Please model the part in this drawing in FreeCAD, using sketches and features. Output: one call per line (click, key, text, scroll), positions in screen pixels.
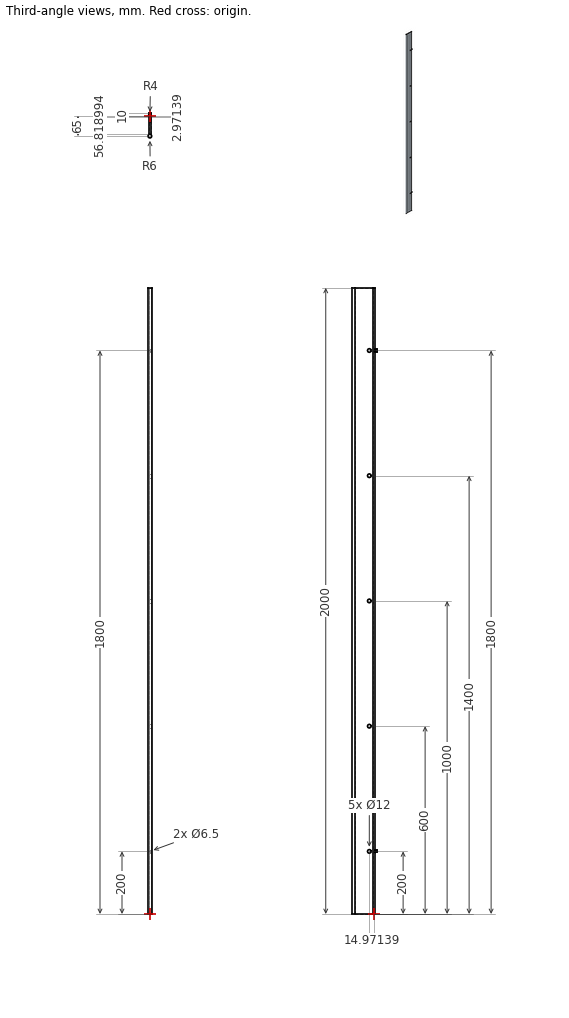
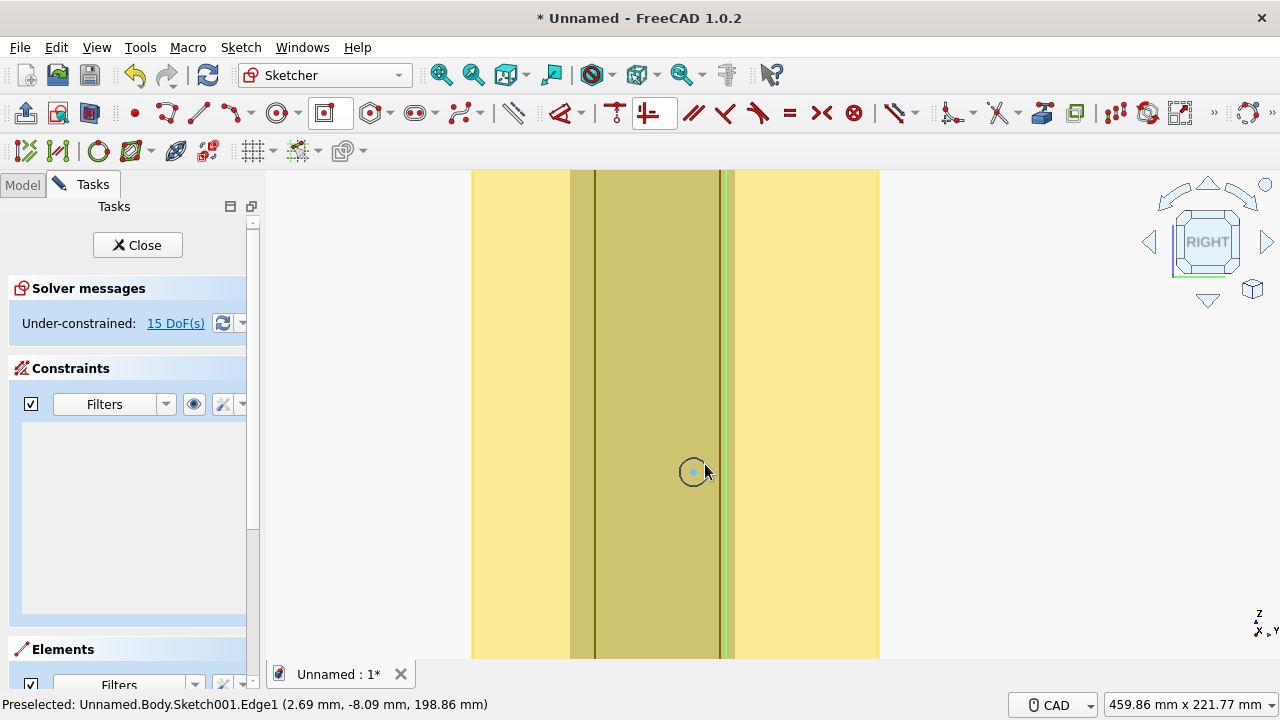
click(703, 462)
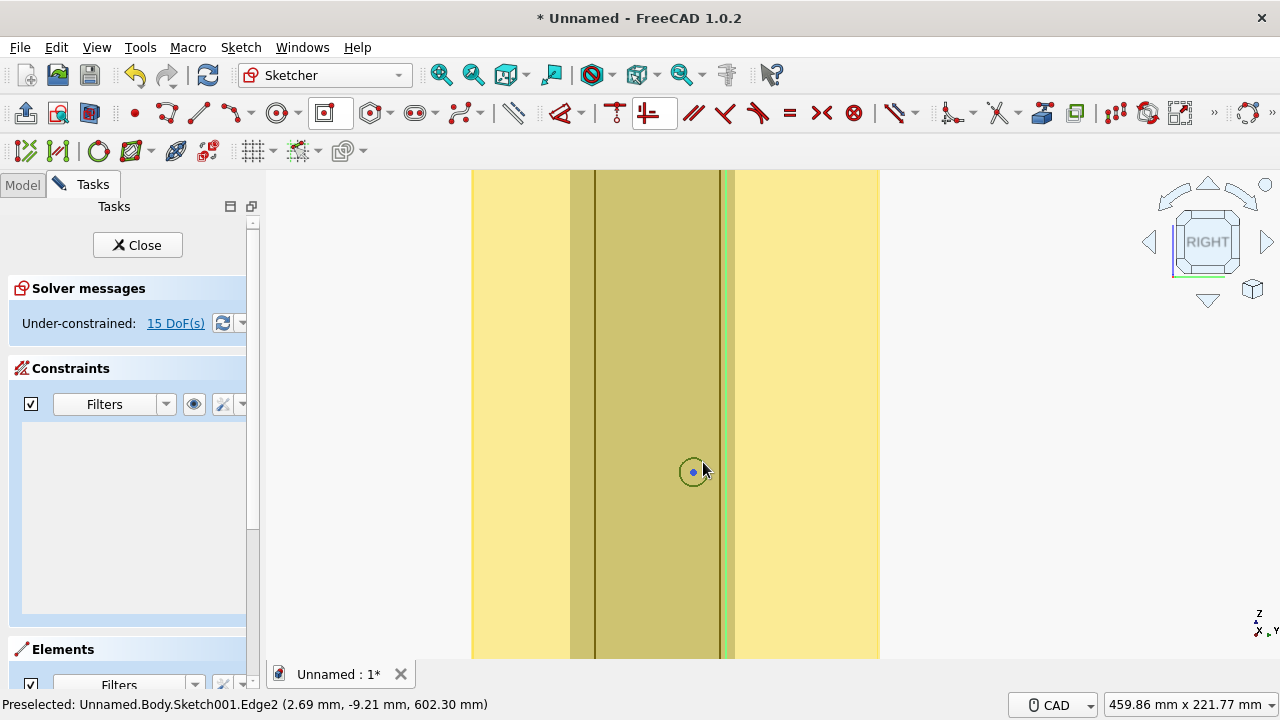
scroll(705, 464, down, 13)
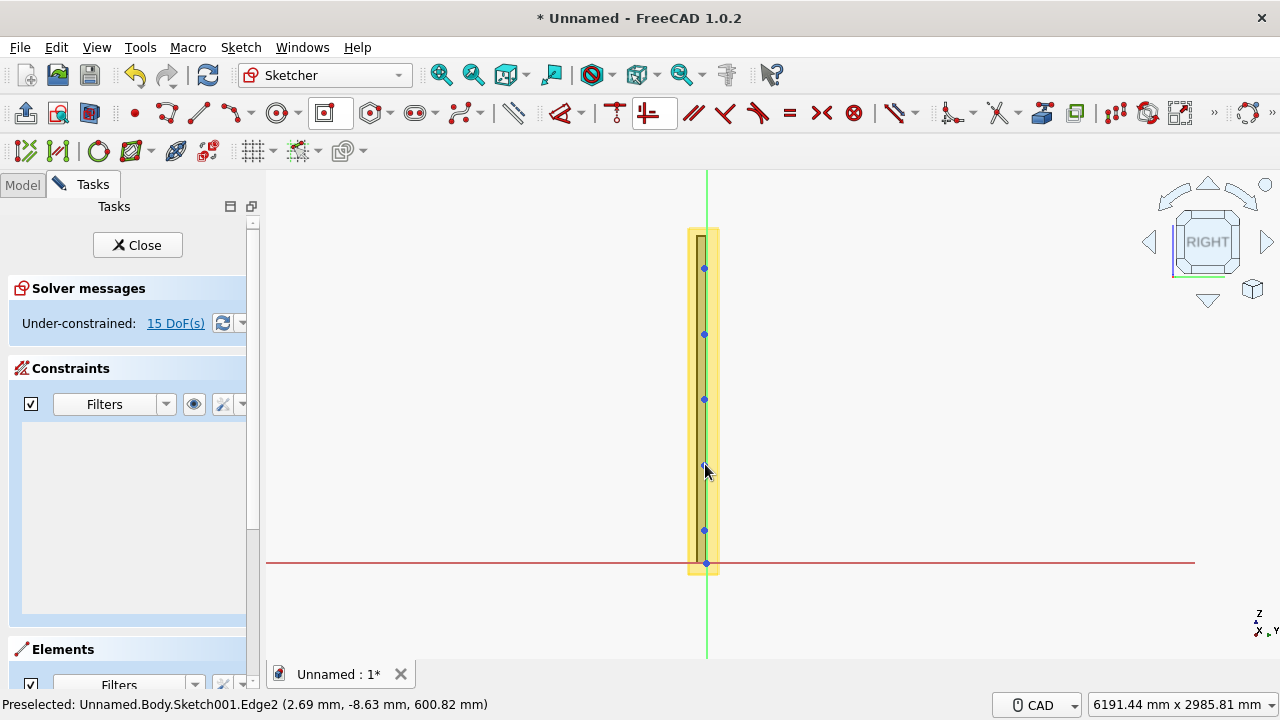
scroll(705, 399, up, 13)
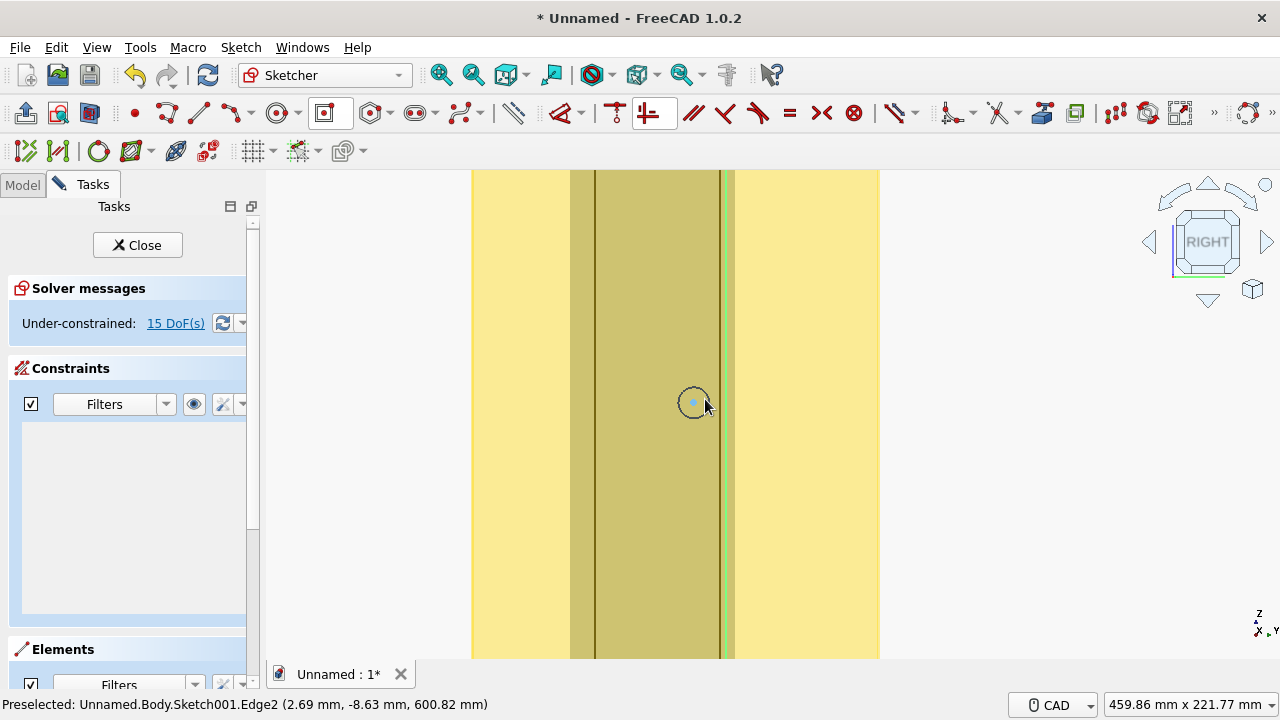
click(705, 392)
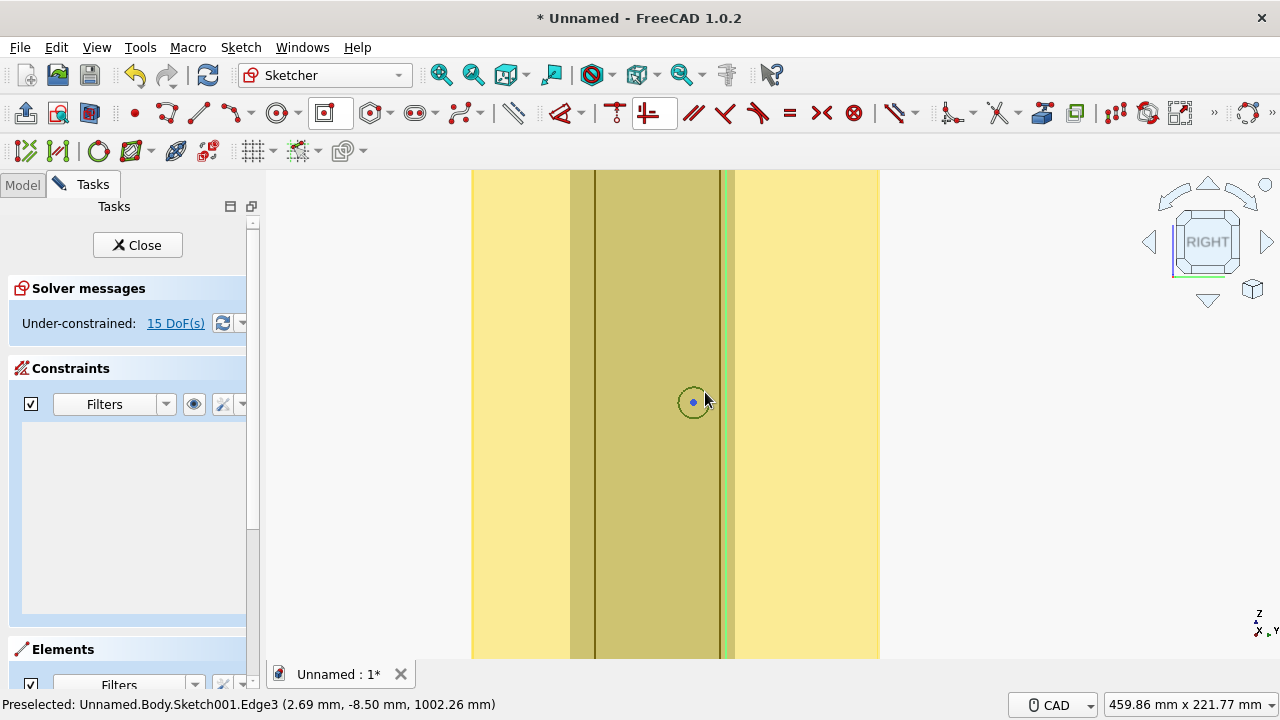
scroll(705, 398, down, 13)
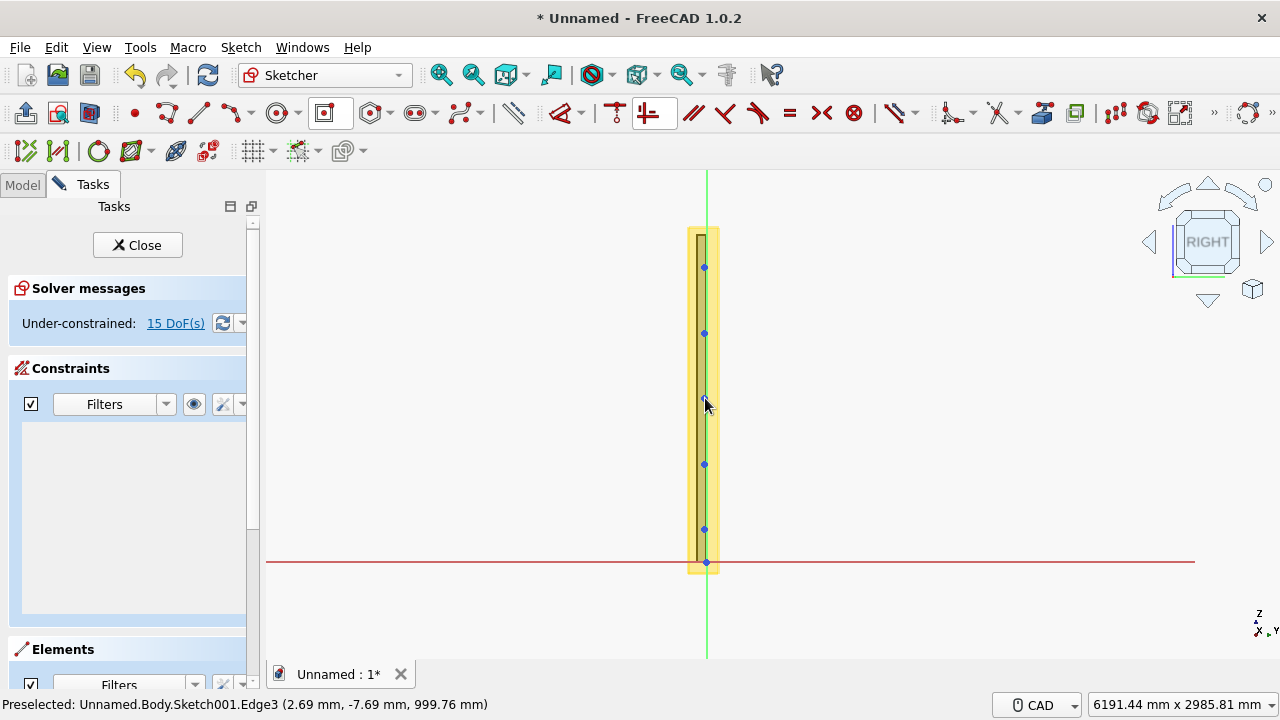
scroll(705, 332, up, 13)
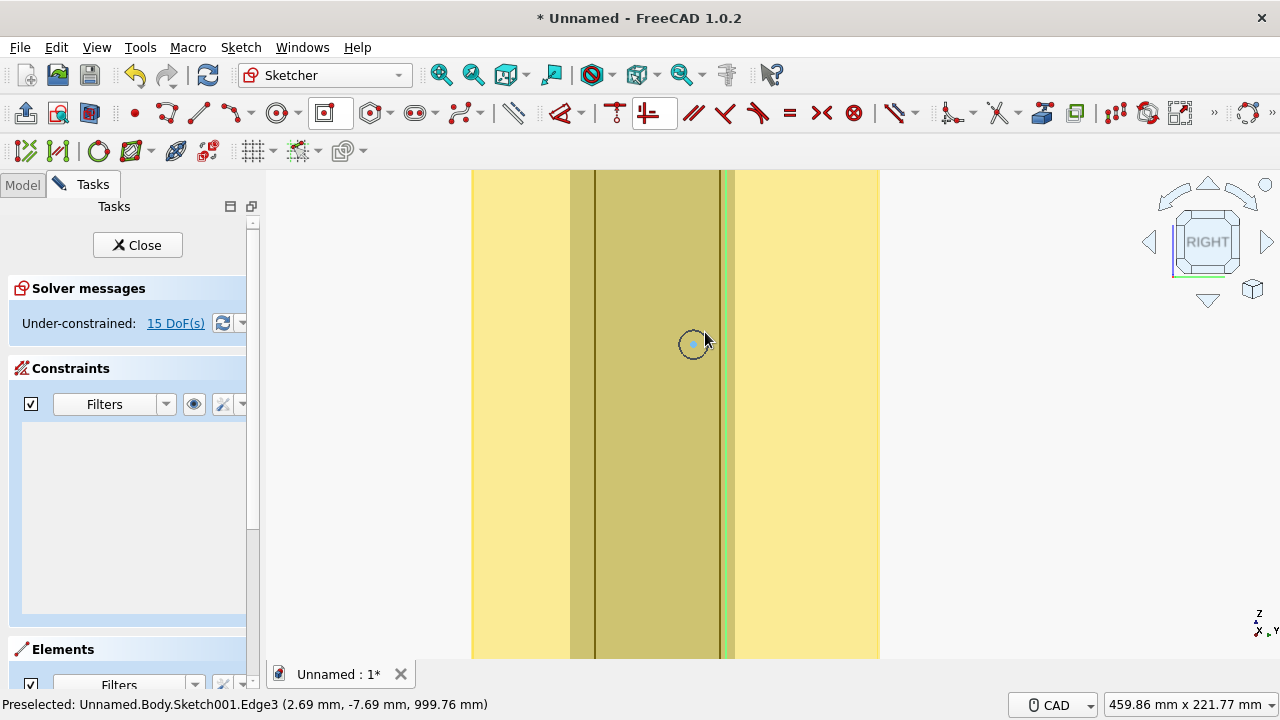
click(704, 335)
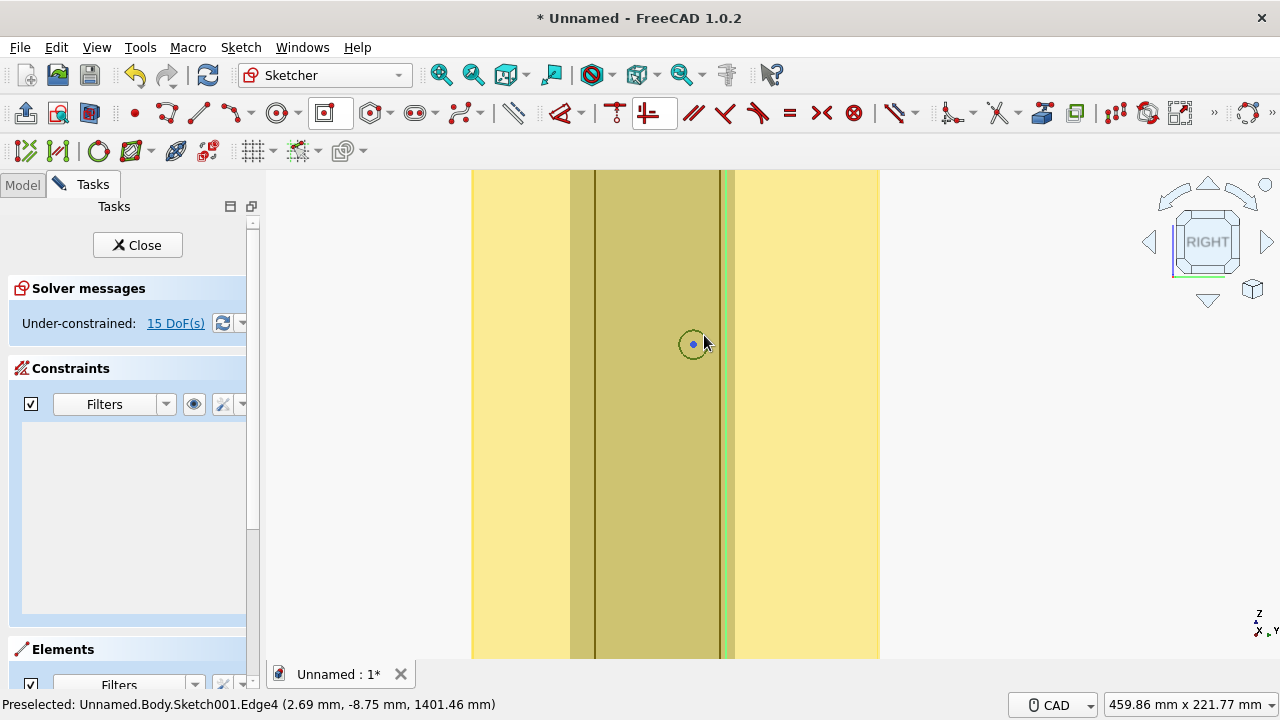
scroll(705, 332, down, 13)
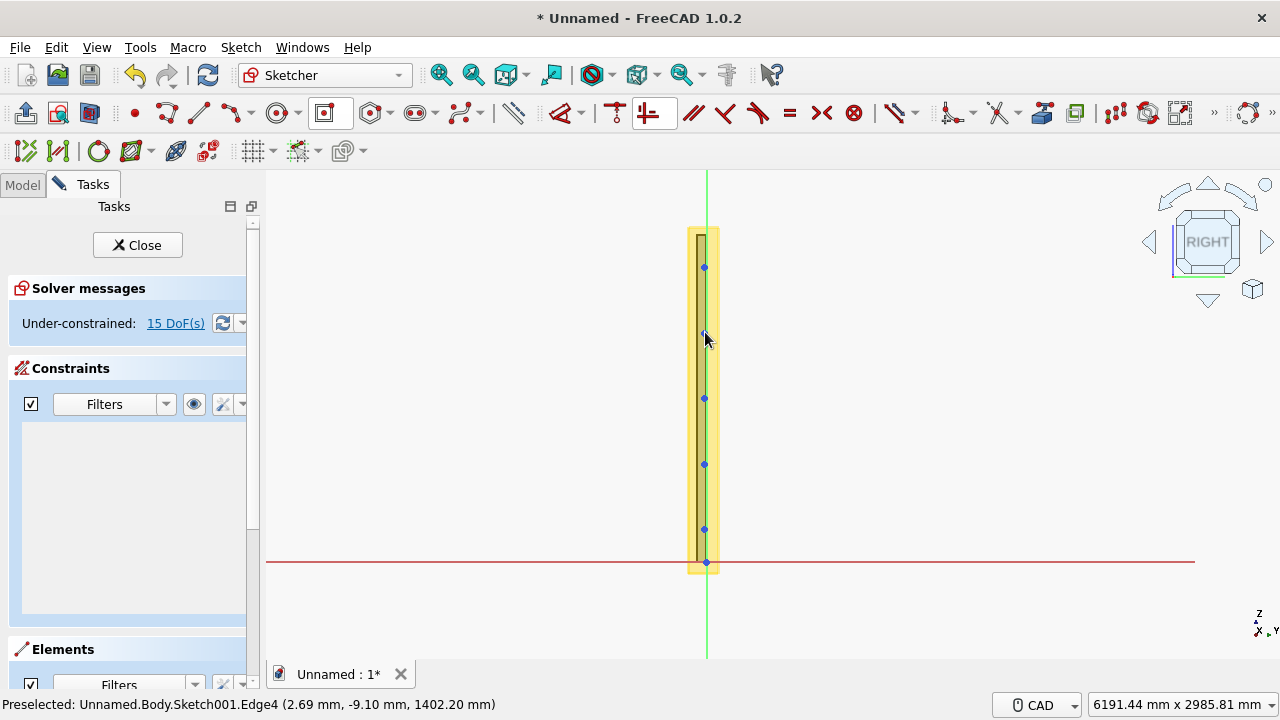
scroll(705, 267, up, 13)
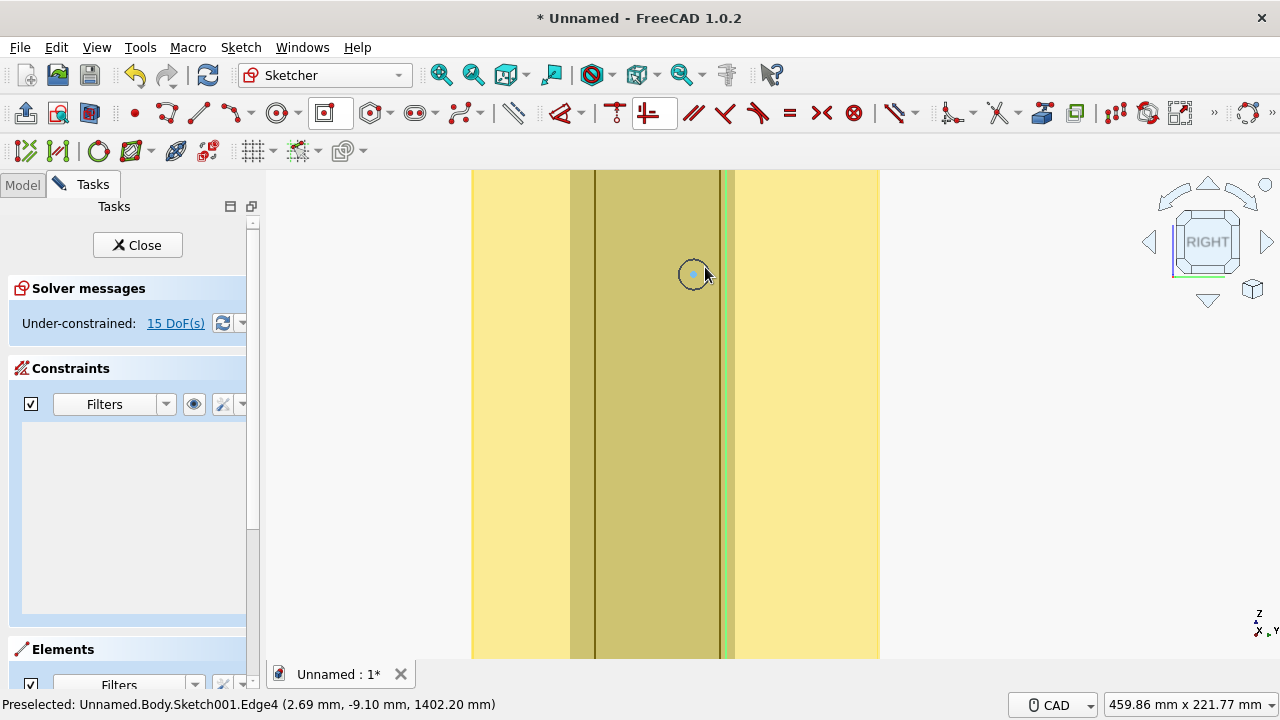
click(705, 264)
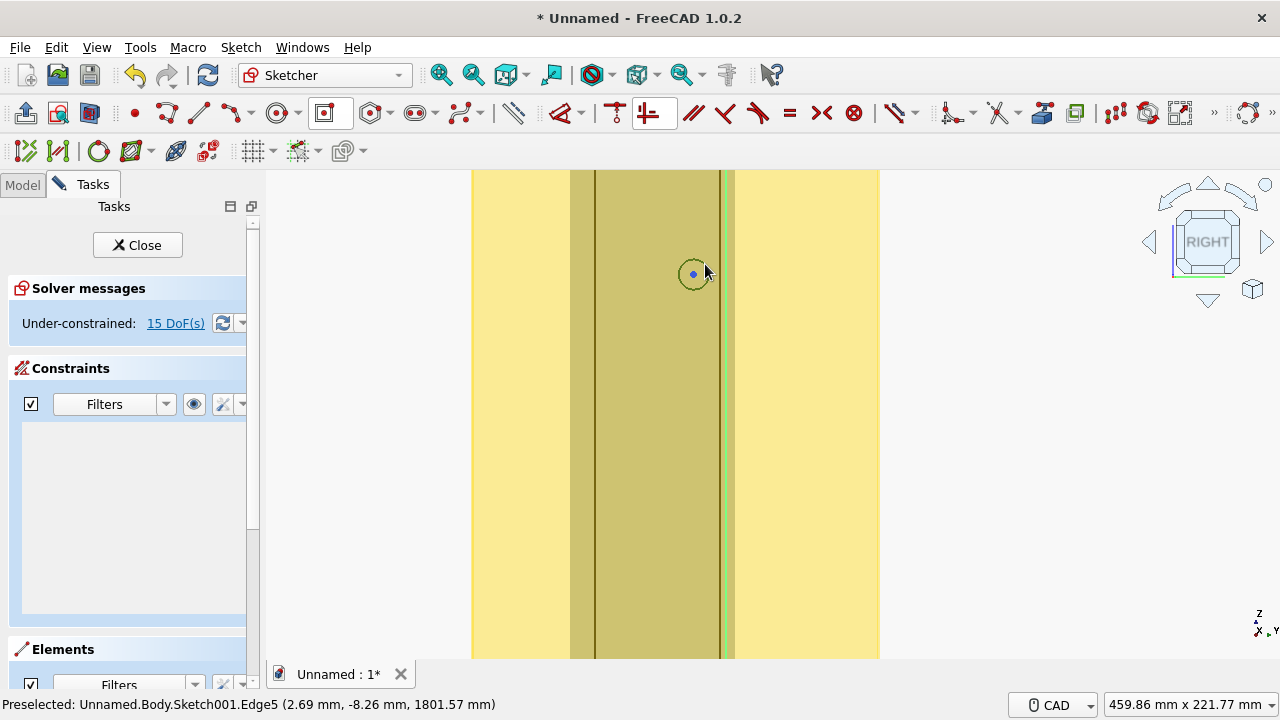
key(e)